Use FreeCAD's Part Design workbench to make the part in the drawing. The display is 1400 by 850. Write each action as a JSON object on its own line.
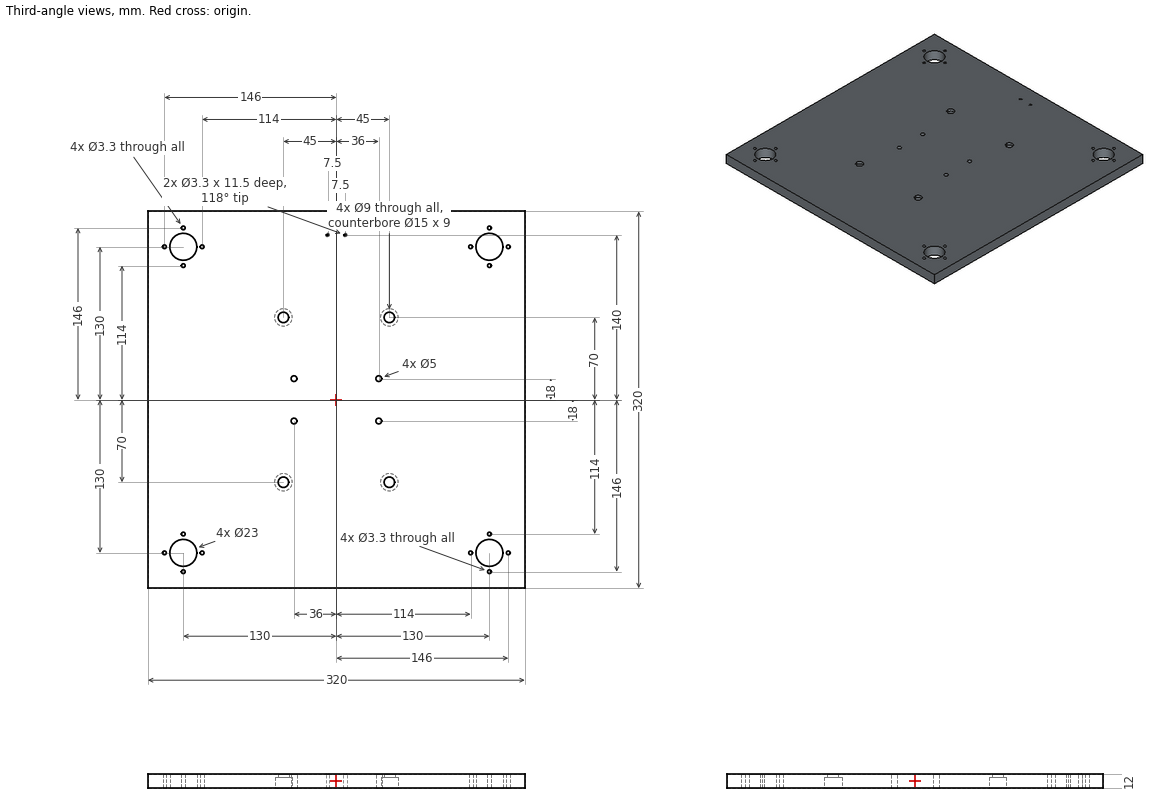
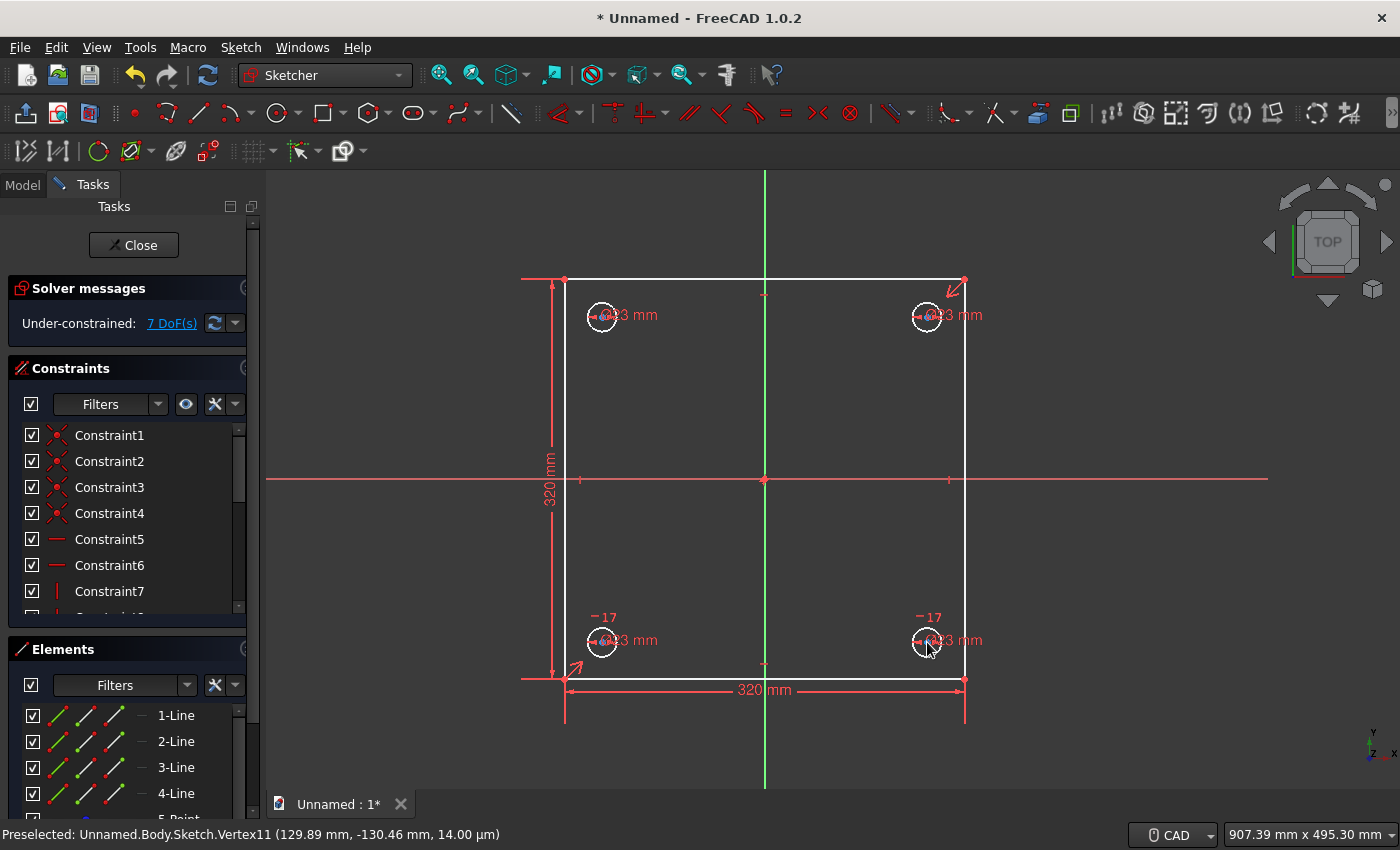
{"action": "left_click", "coordinate": [602, 642]}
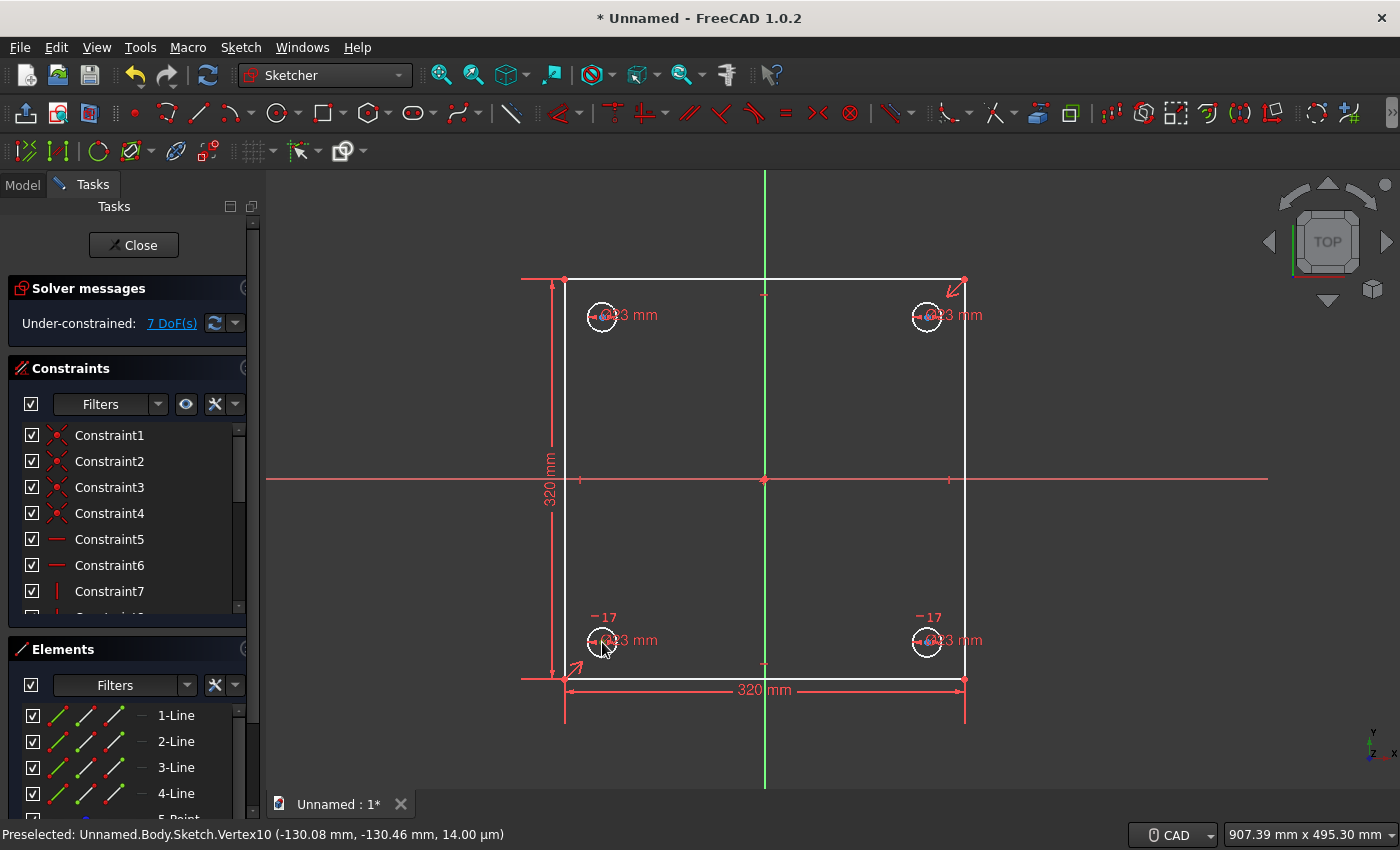
{"action": "left_click", "coordinate": [602, 317]}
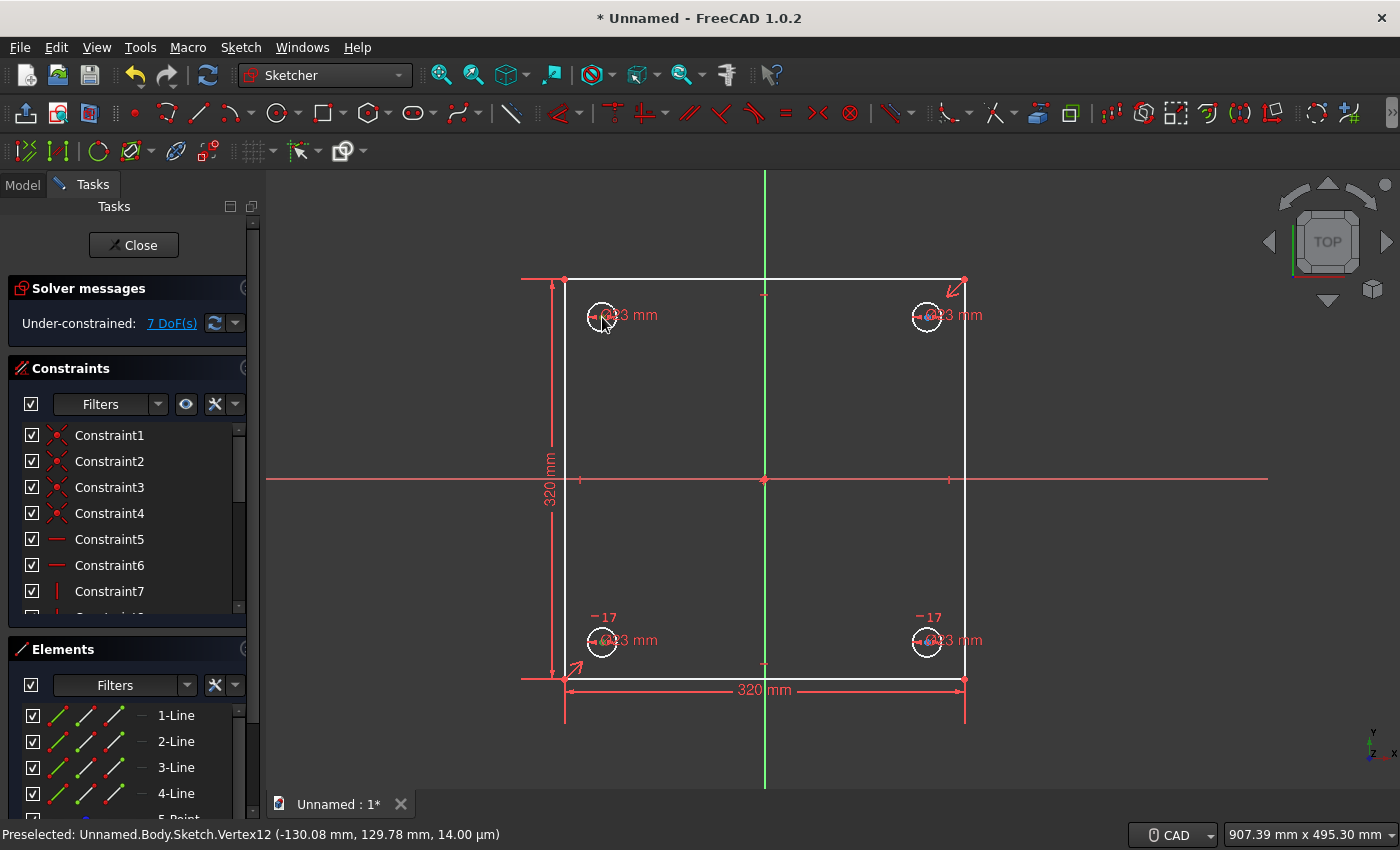
{"action": "left_click", "coordinate": [668, 114]}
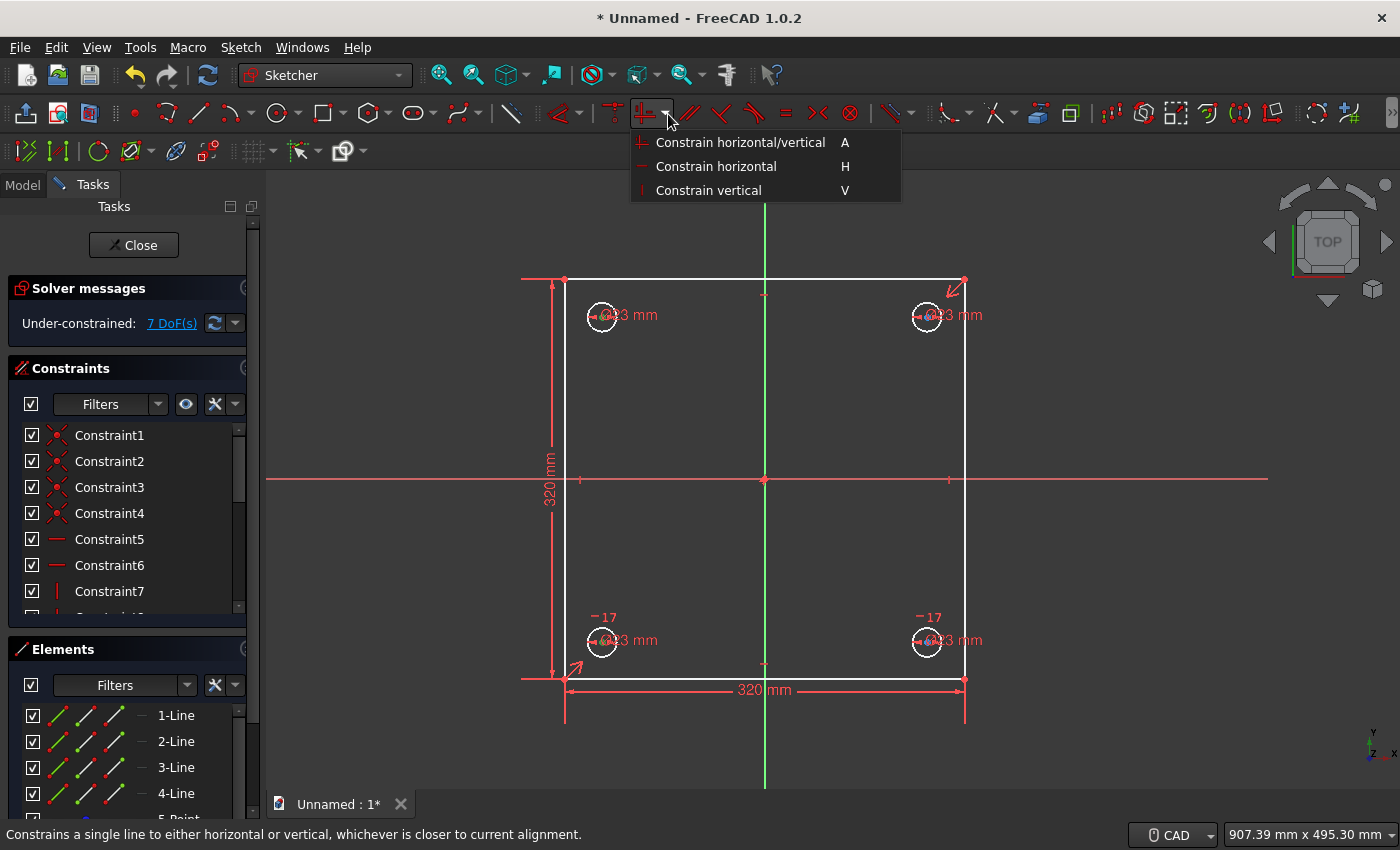
{"action": "left_click", "coordinate": [766, 190]}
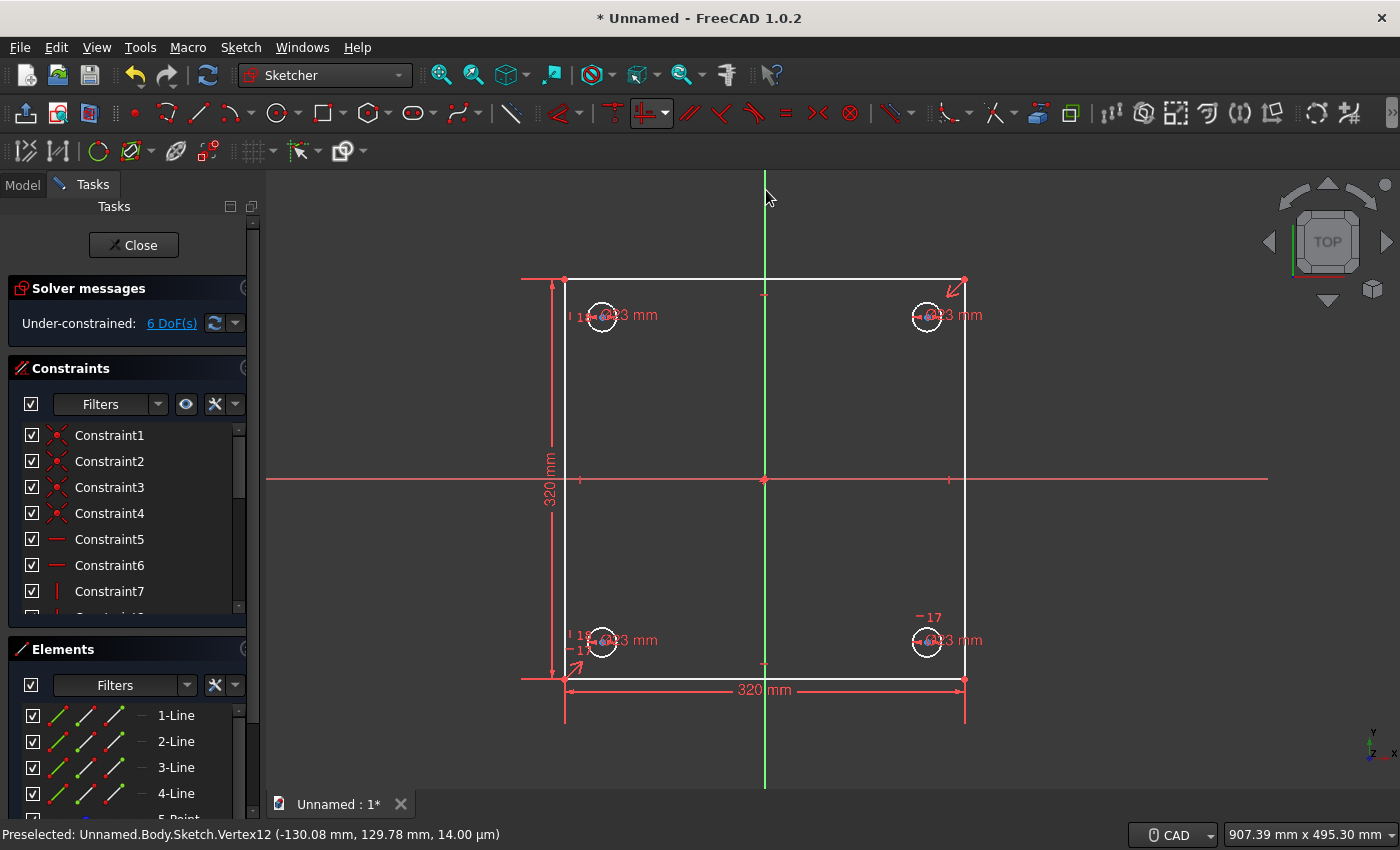
{"action": "left_click", "coordinate": [927, 642]}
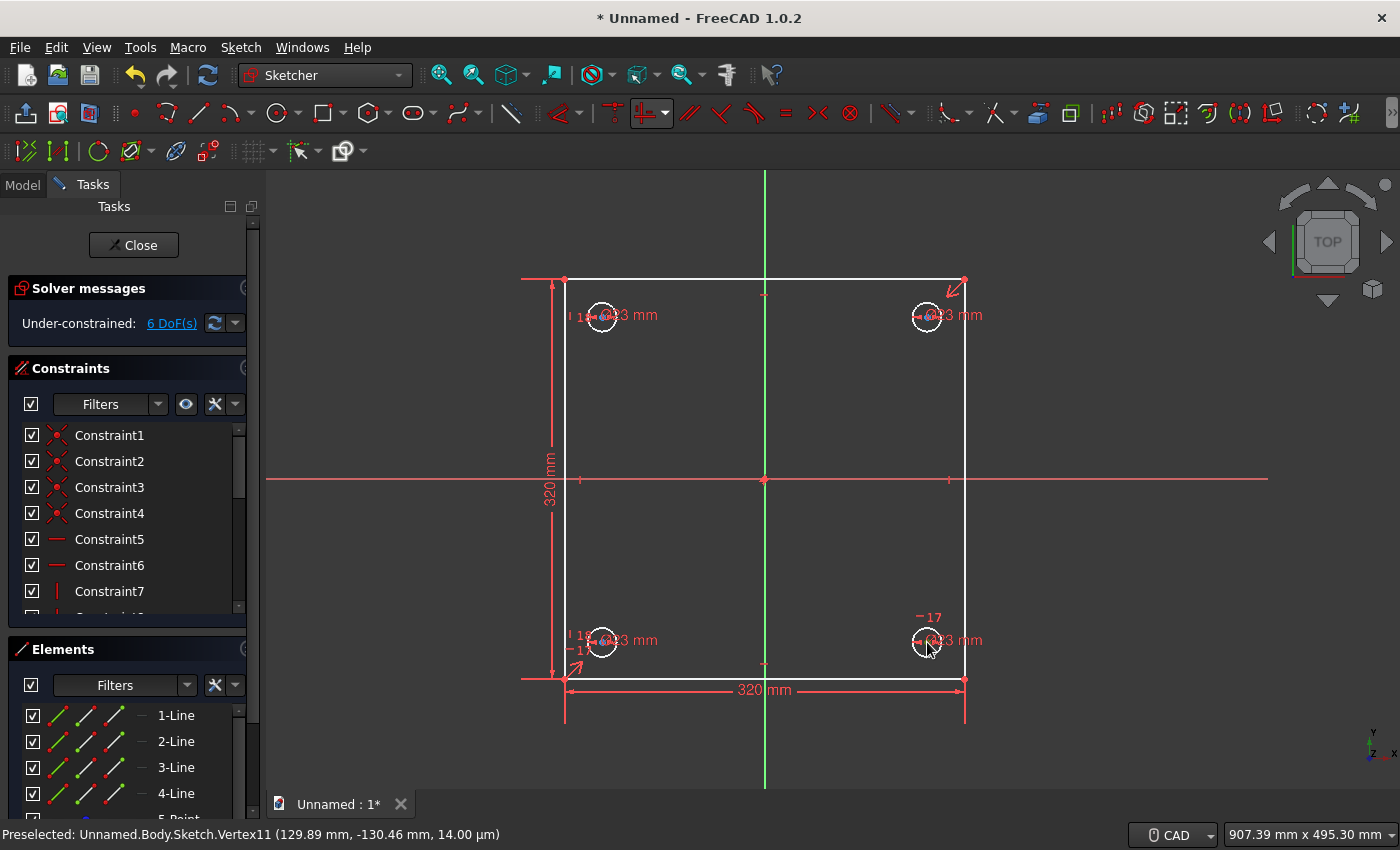
{"action": "left_click", "coordinate": [927, 317]}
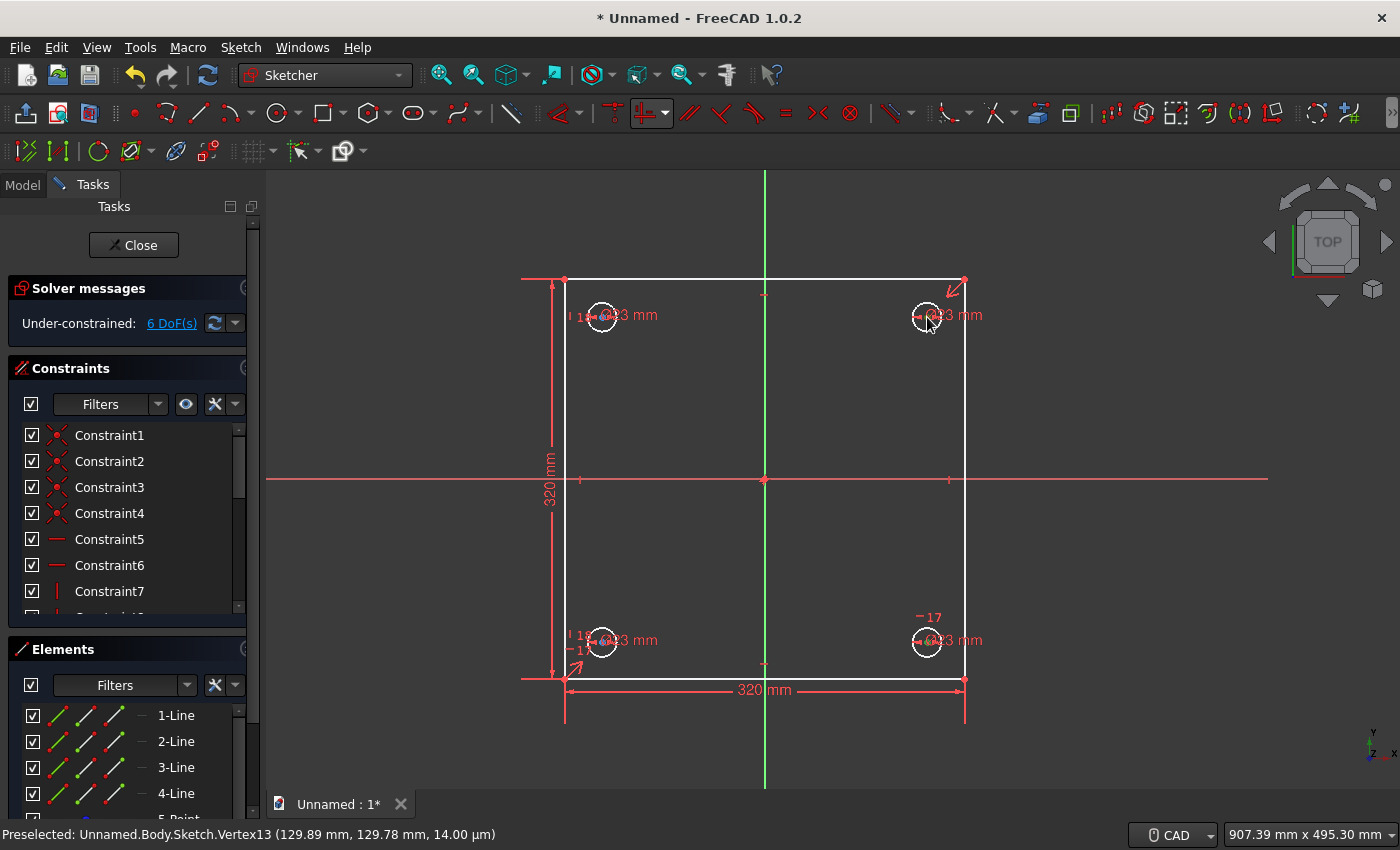
{"action": "key", "text": "v"}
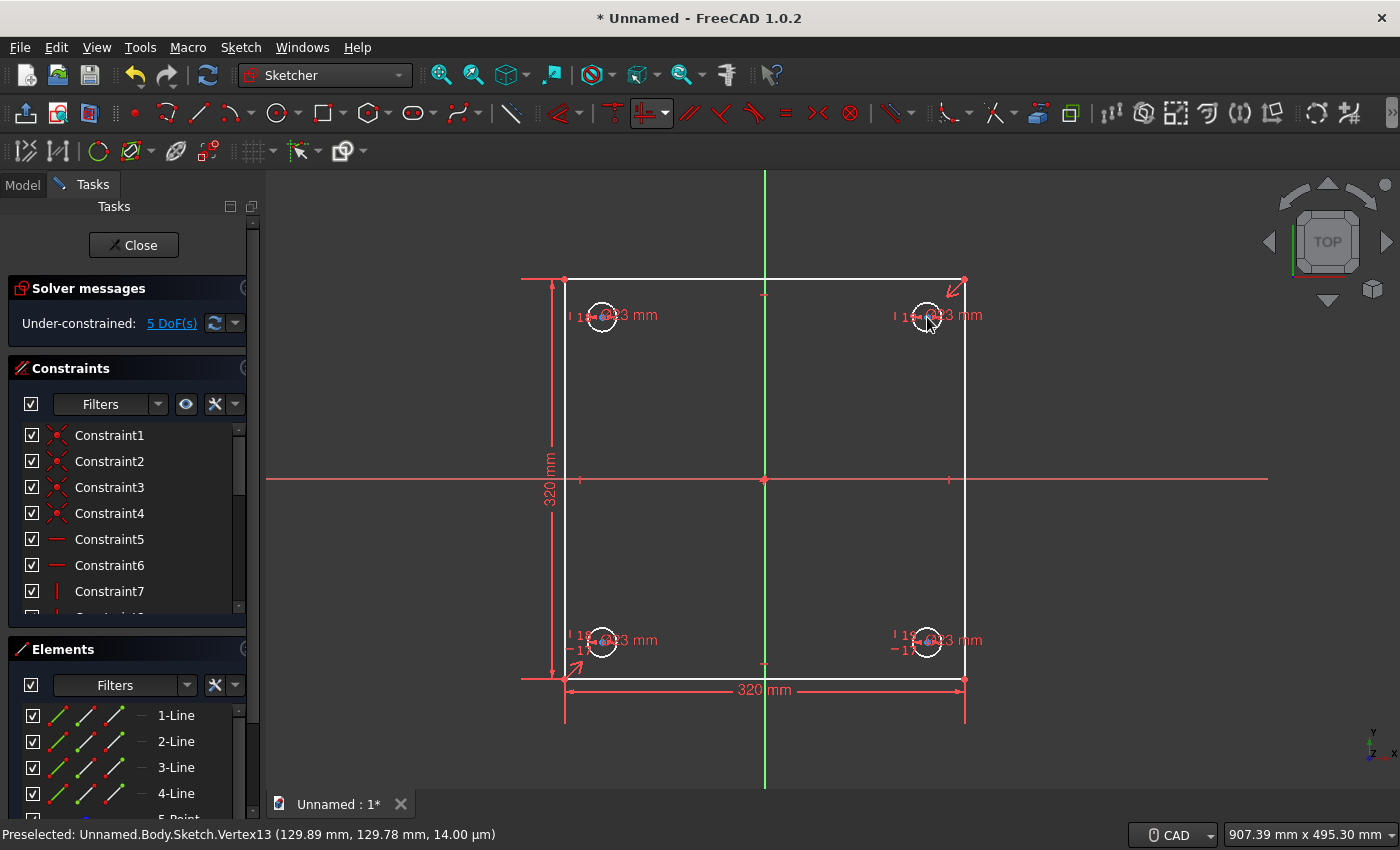
{"action": "left_click", "coordinate": [602, 317]}